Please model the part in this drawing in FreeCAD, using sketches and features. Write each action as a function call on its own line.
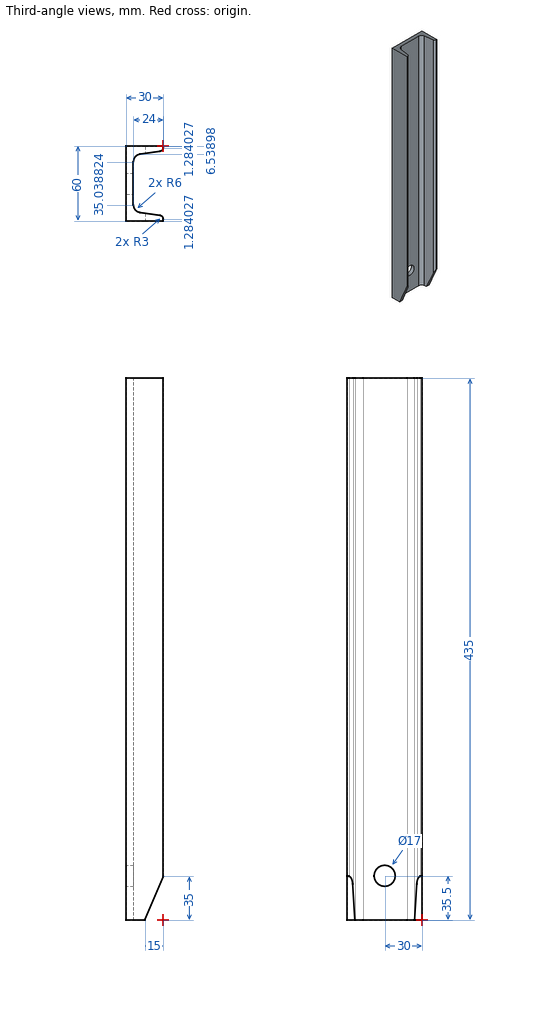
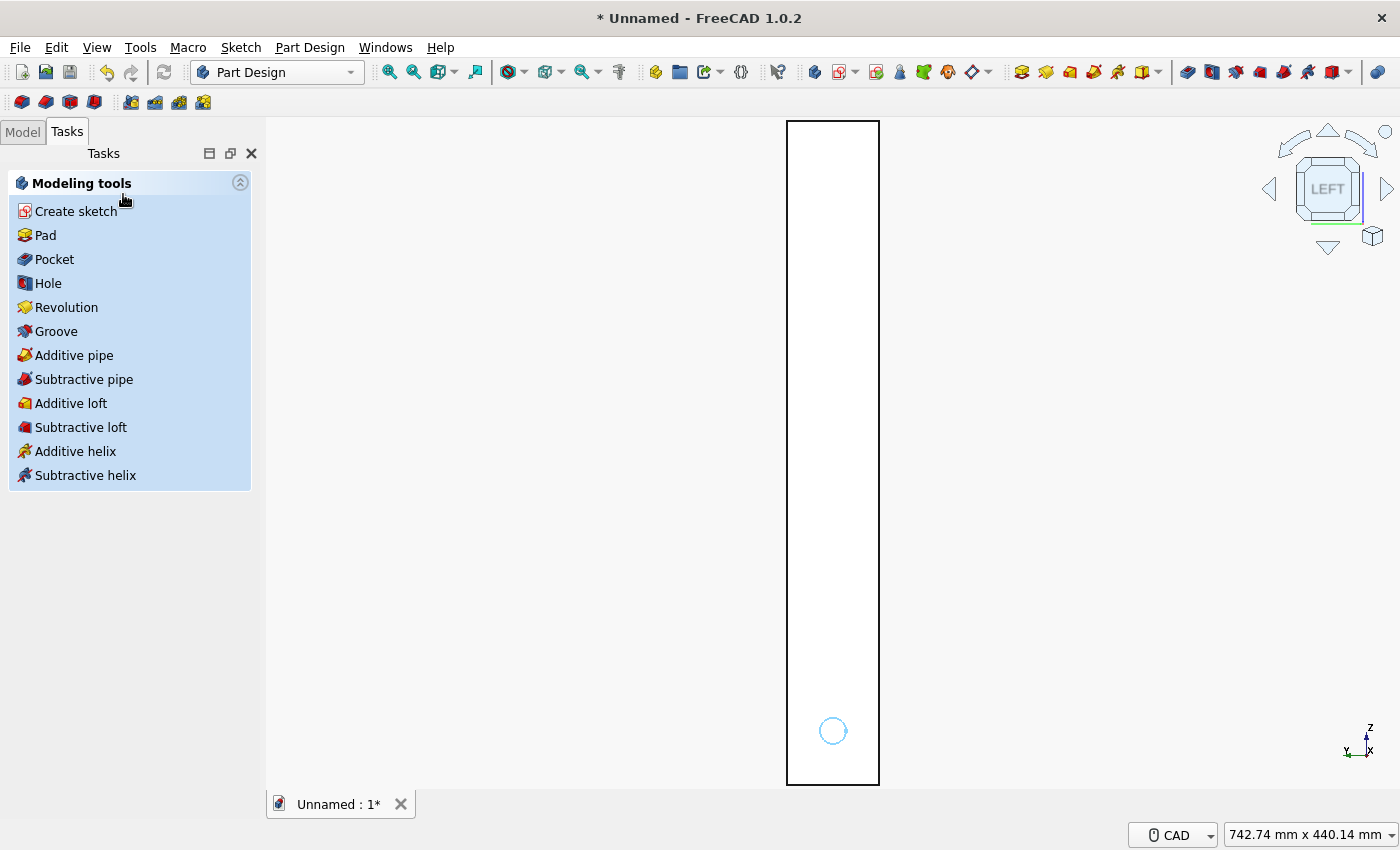
click(1188, 72)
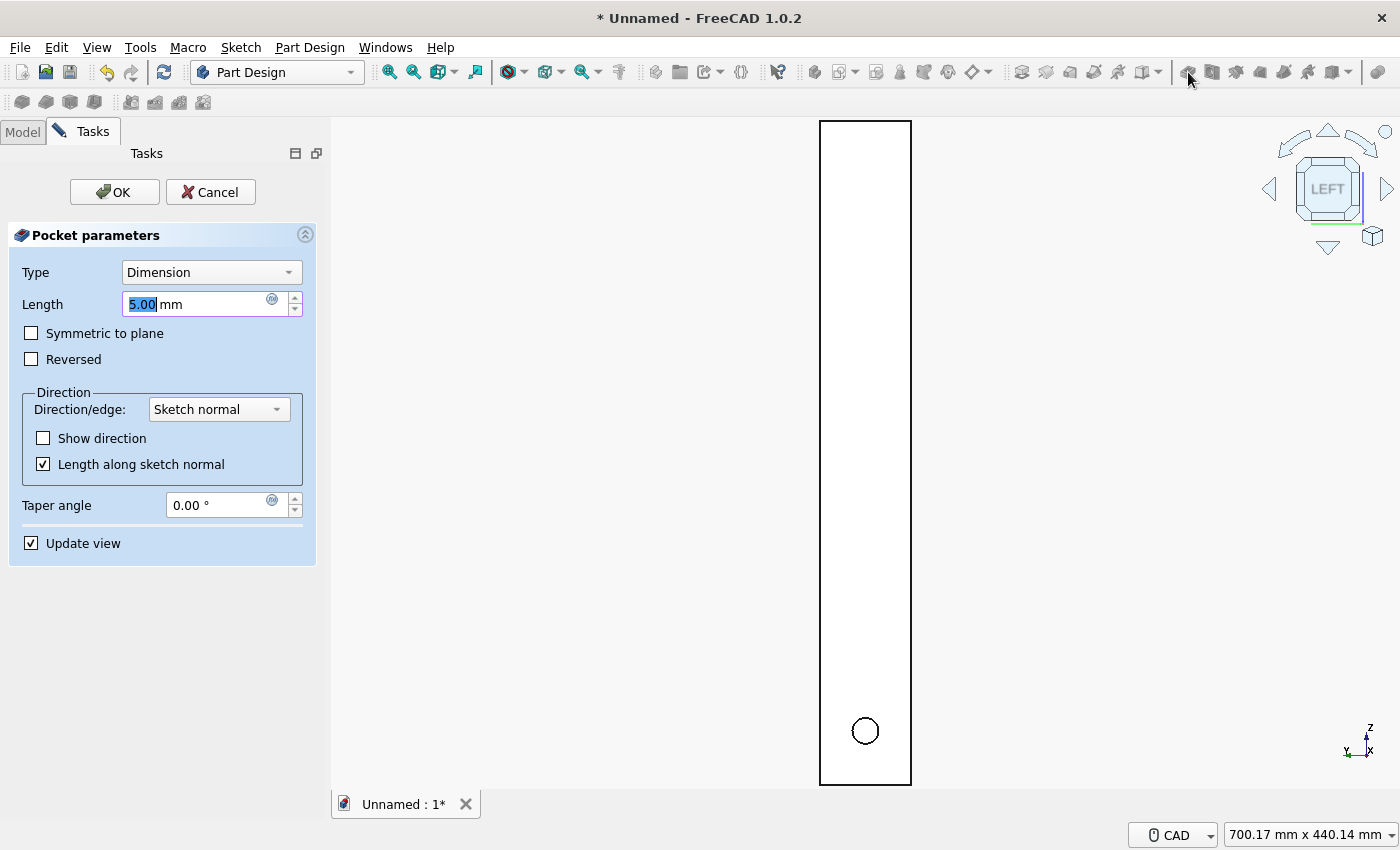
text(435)
key(Tab)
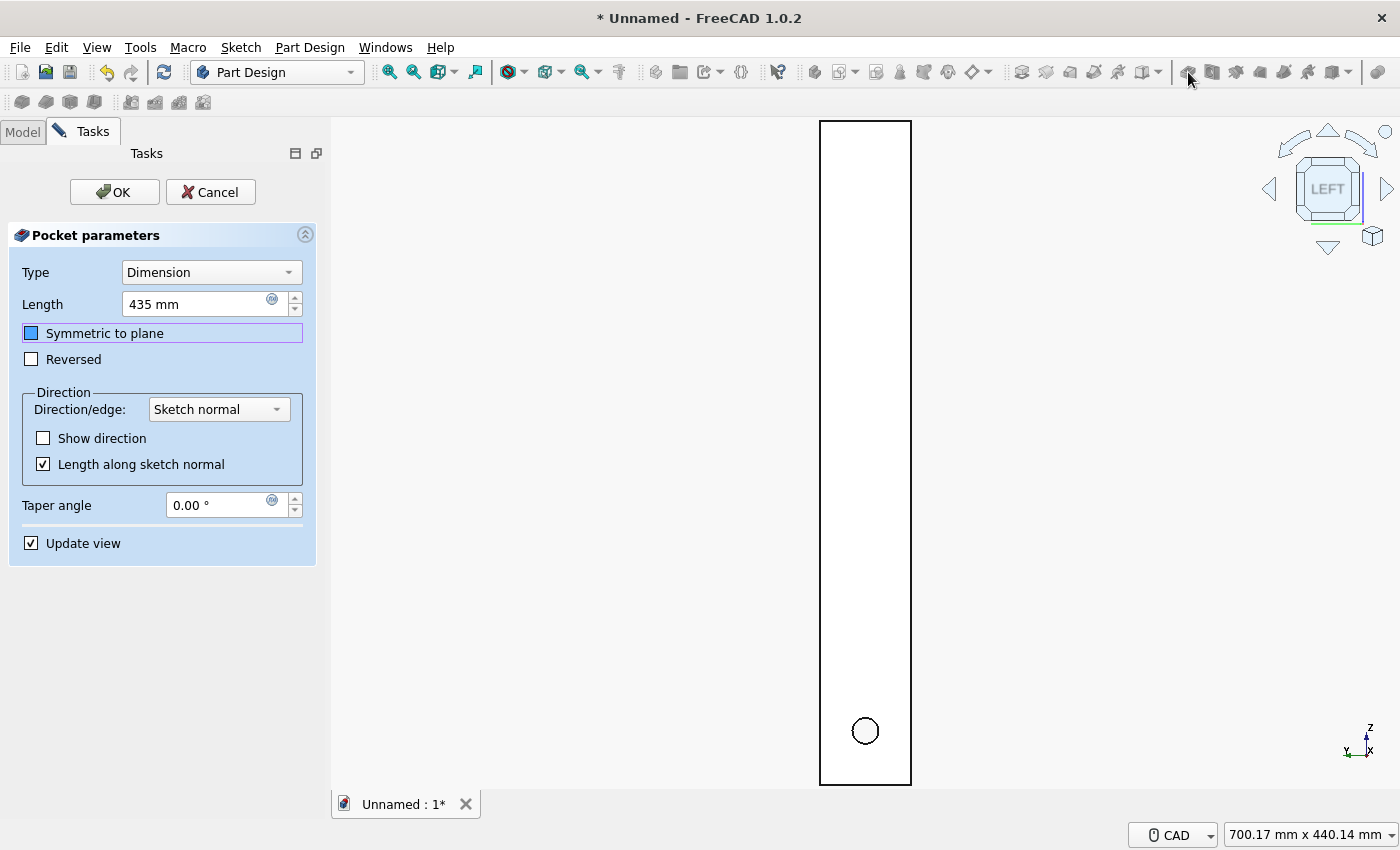
click(115, 192)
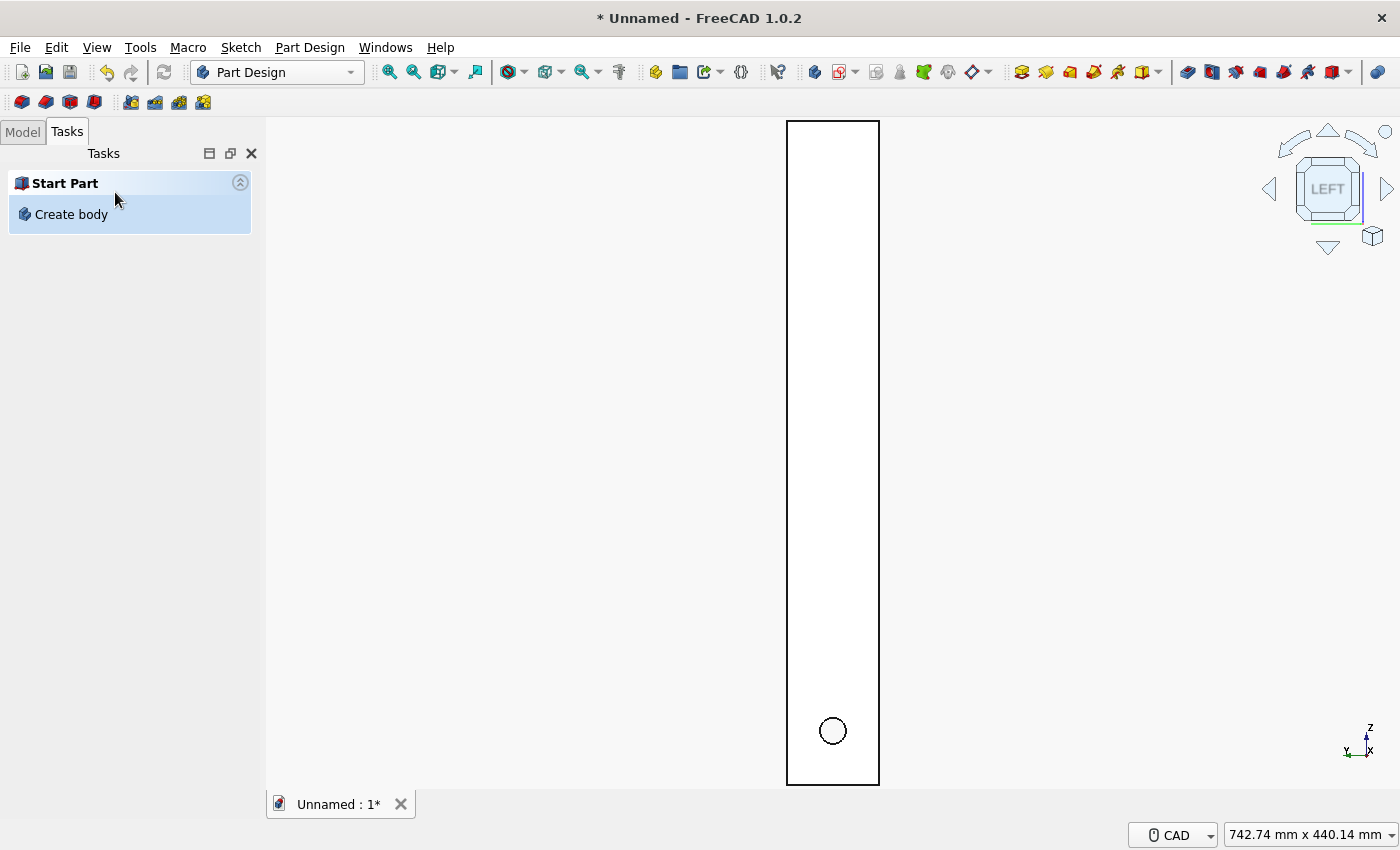
key(4)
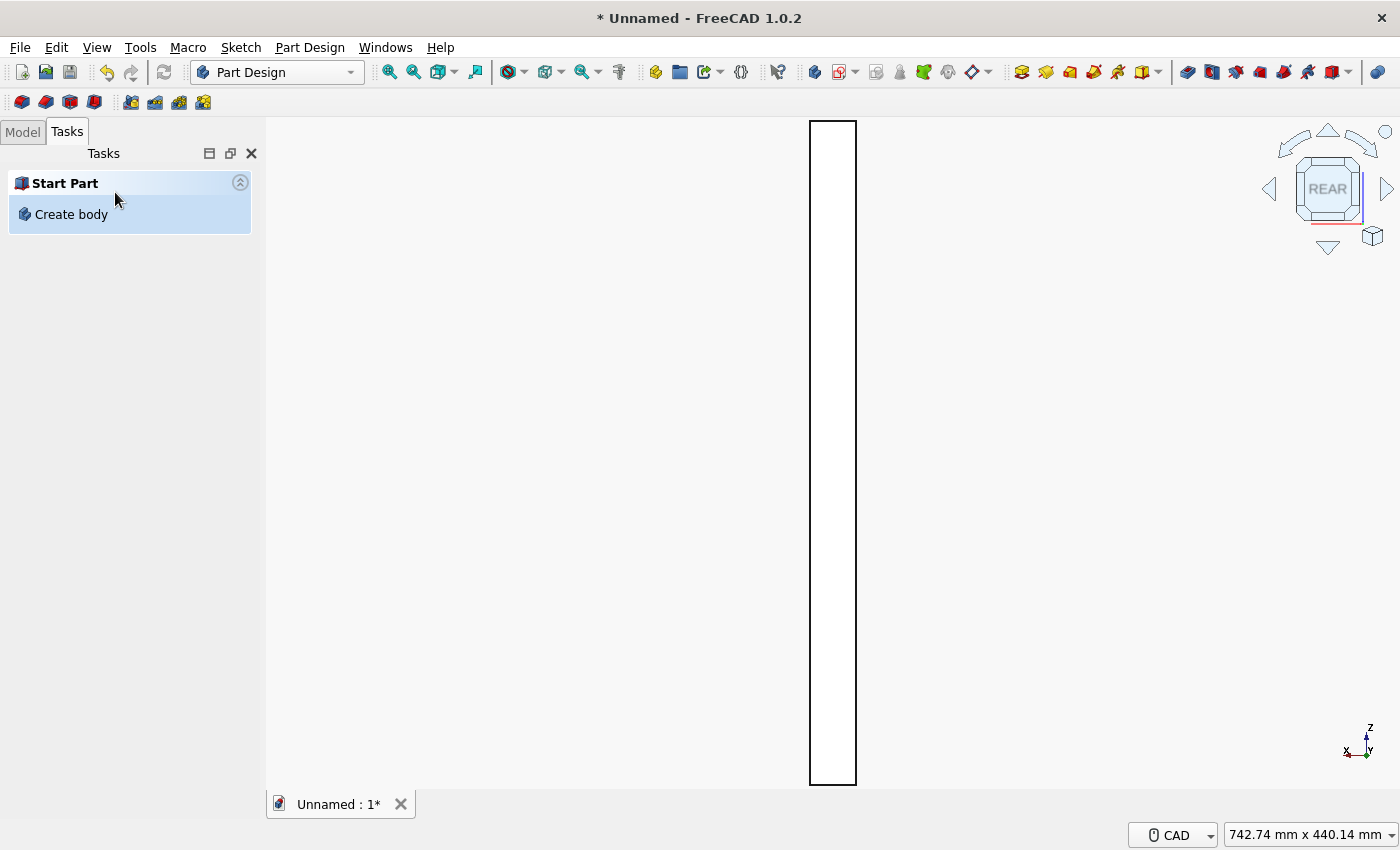
click(833, 167)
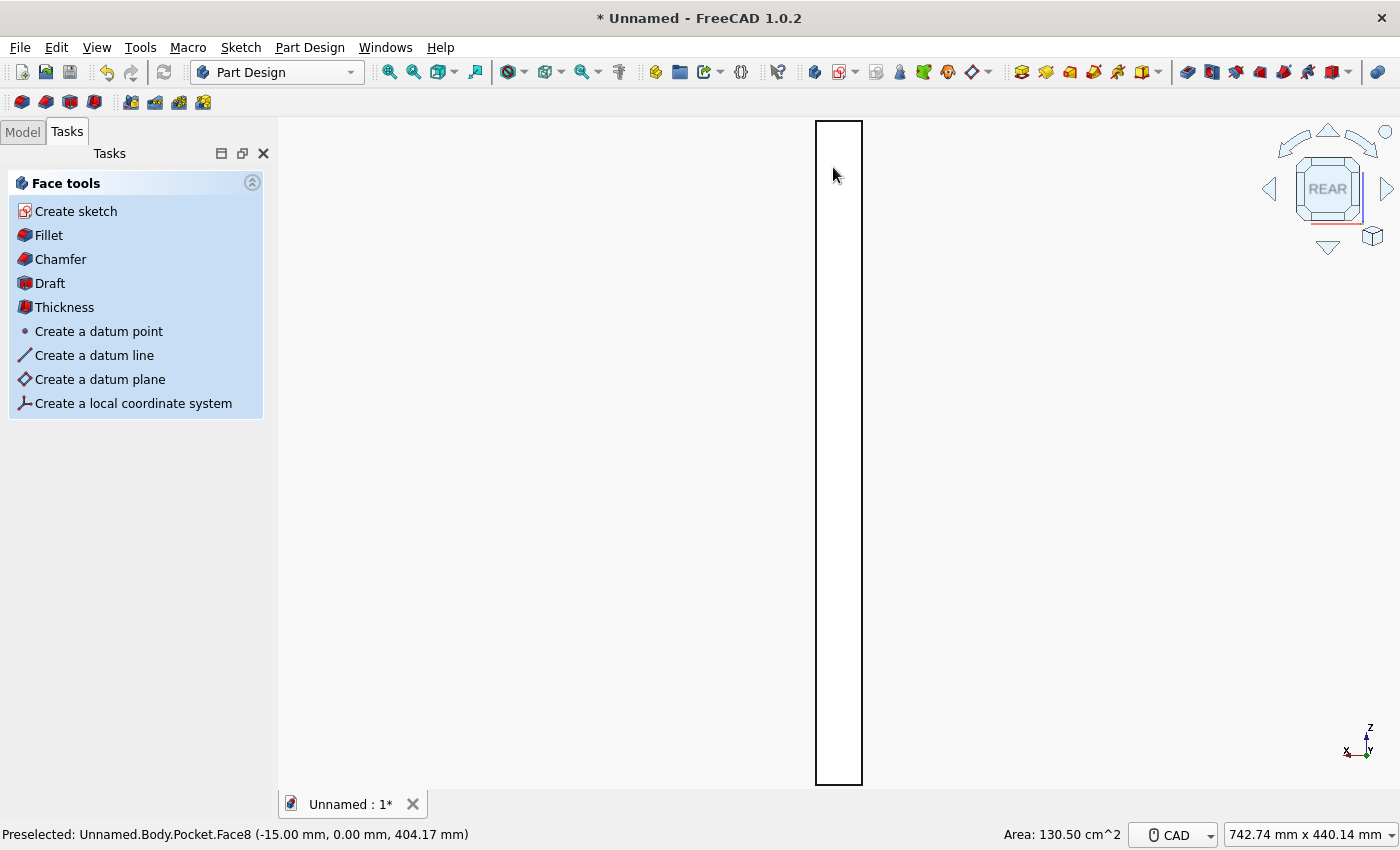
click(840, 72)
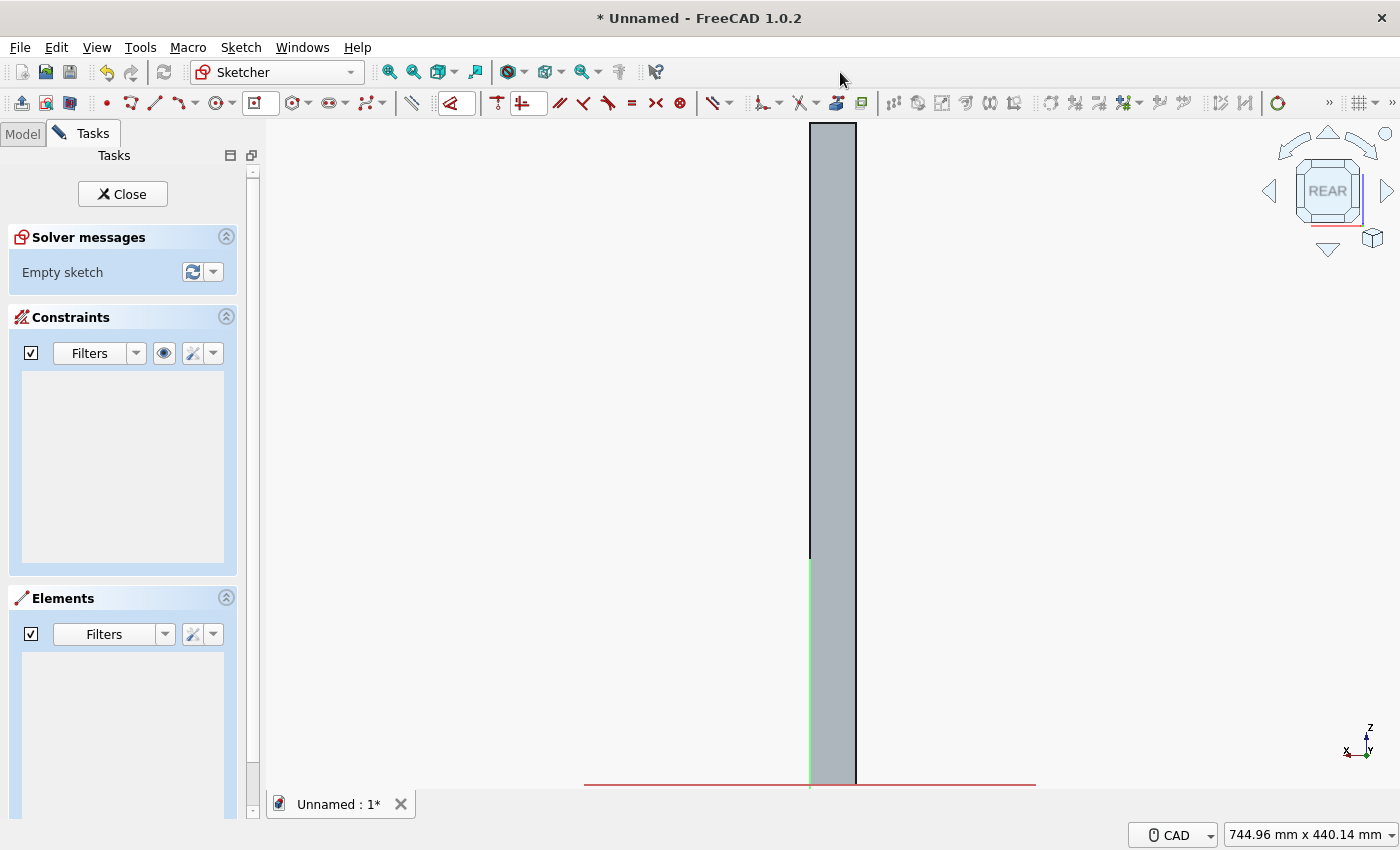
scroll(764, 454, down, 5)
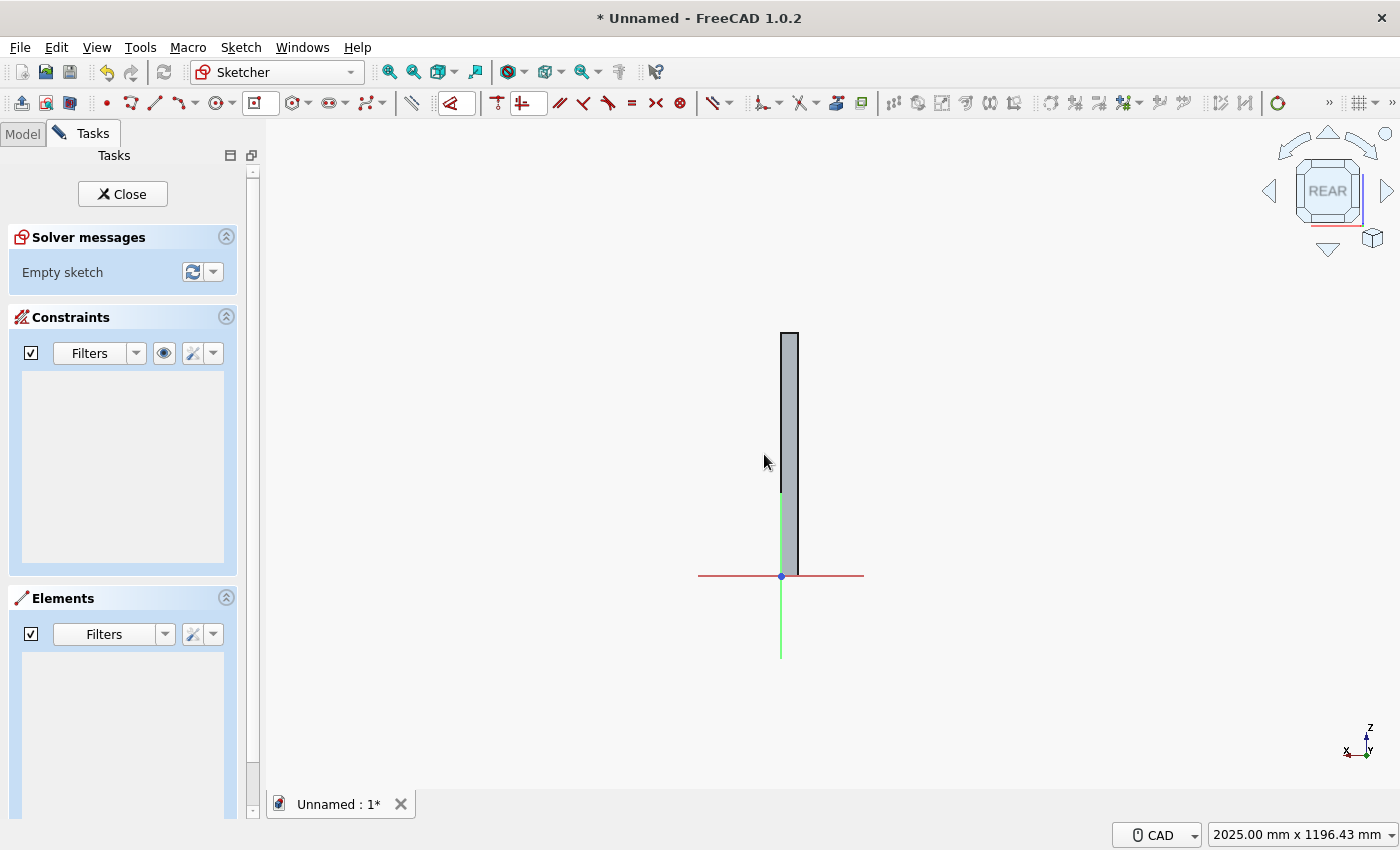
scroll(787, 572, up, 15)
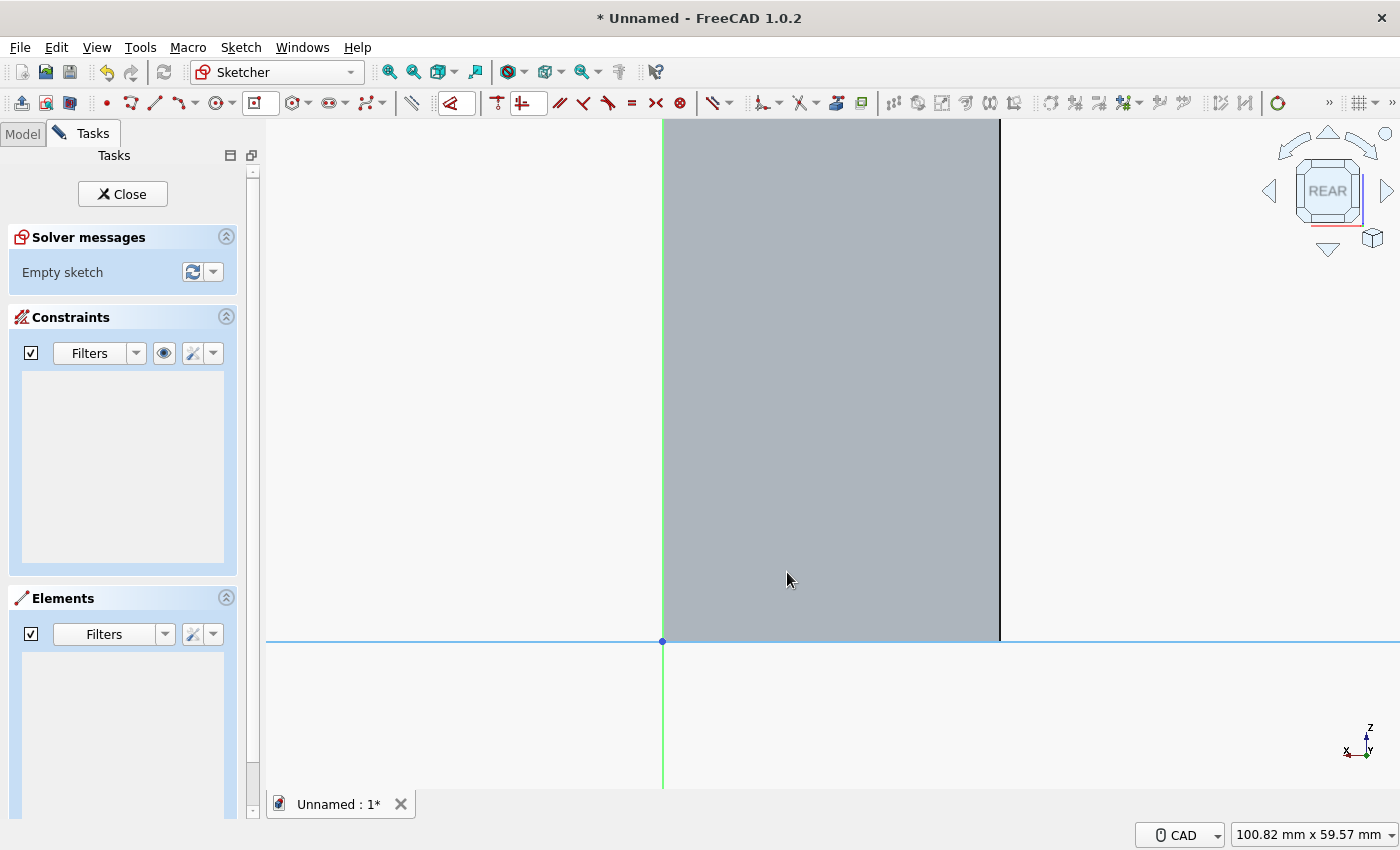
click(132, 104)